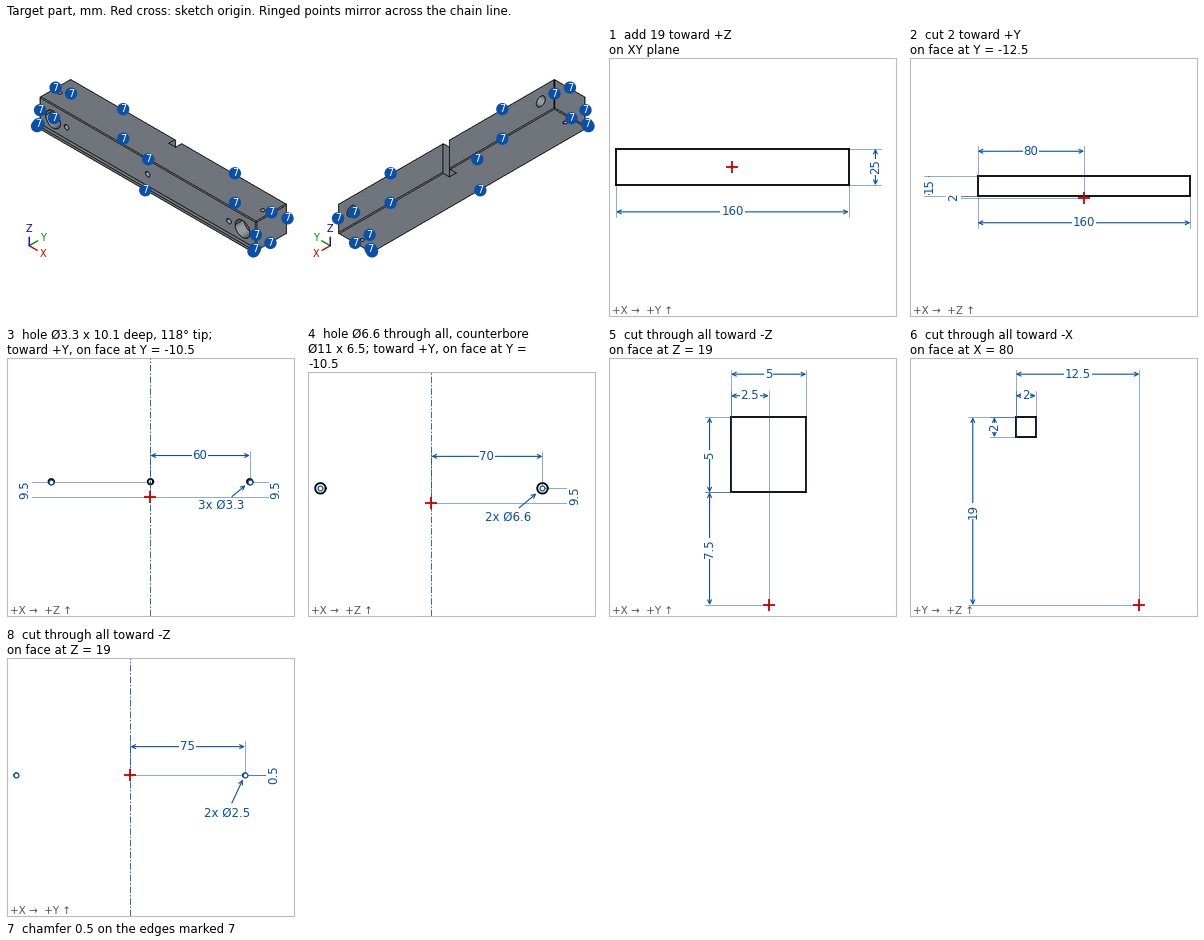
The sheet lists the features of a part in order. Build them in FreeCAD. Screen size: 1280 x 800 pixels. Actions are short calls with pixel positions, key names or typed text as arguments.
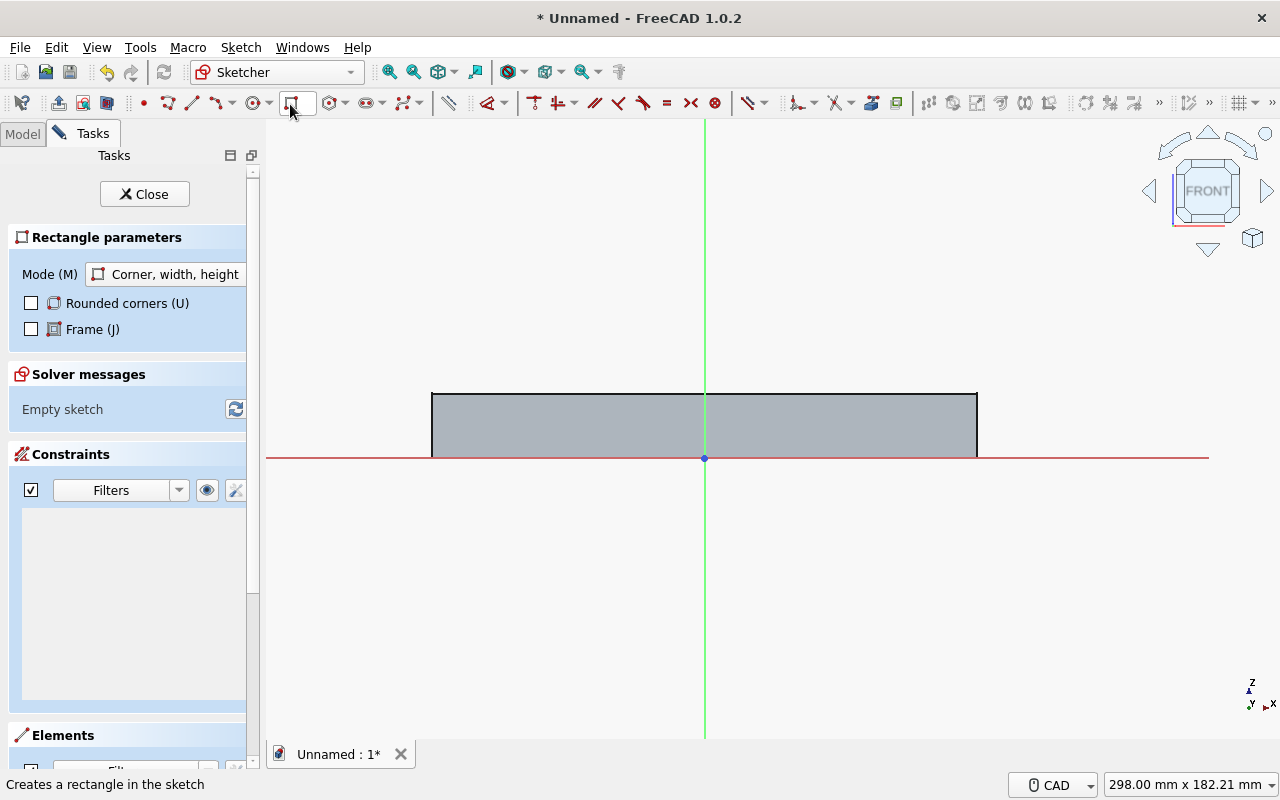
click(432, 400)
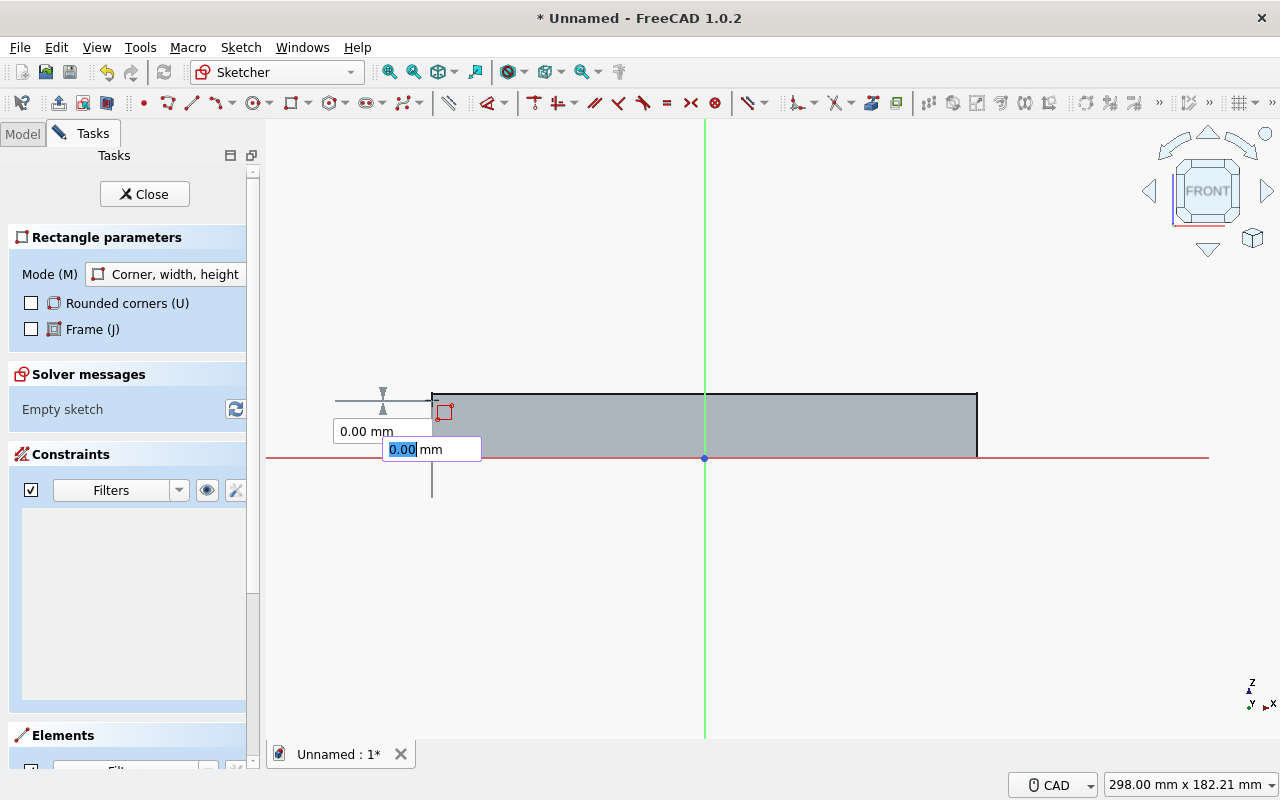
scroll(977, 451, up, 5)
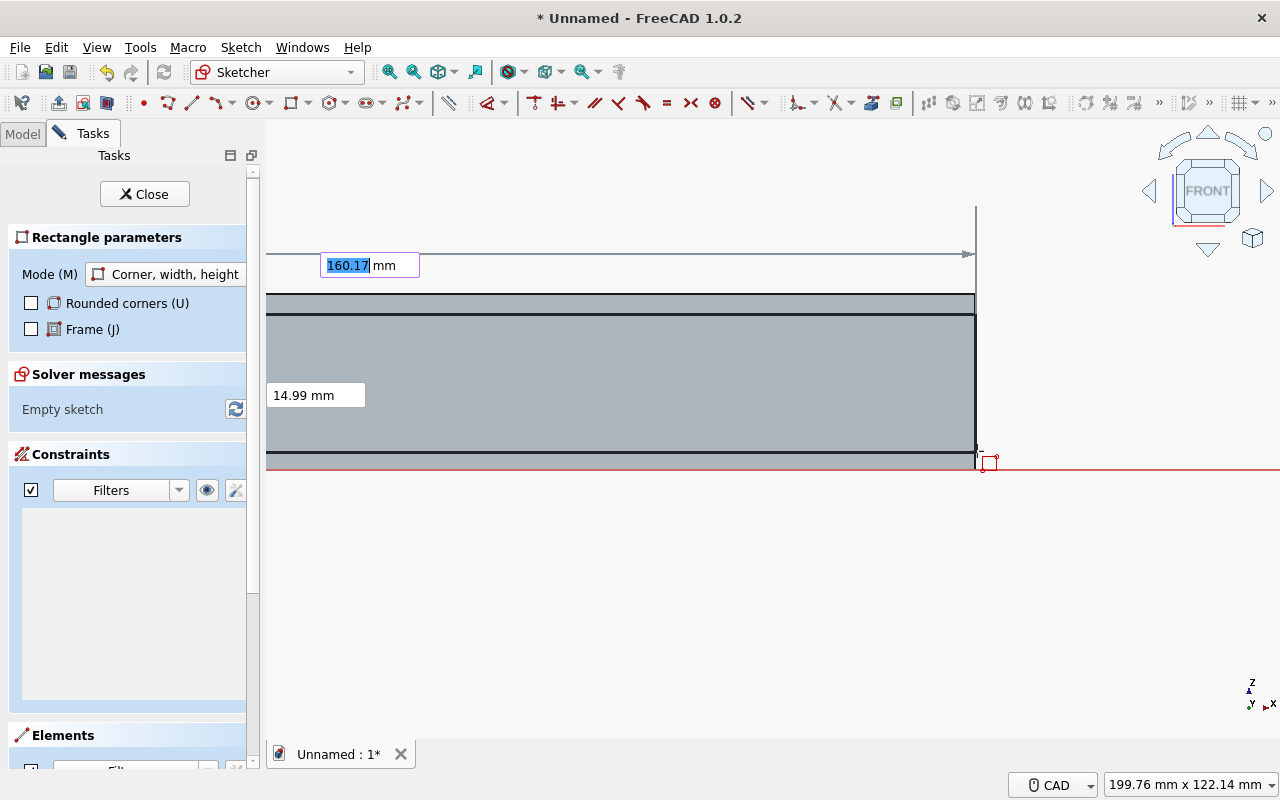
click(975, 451)
key(Escape)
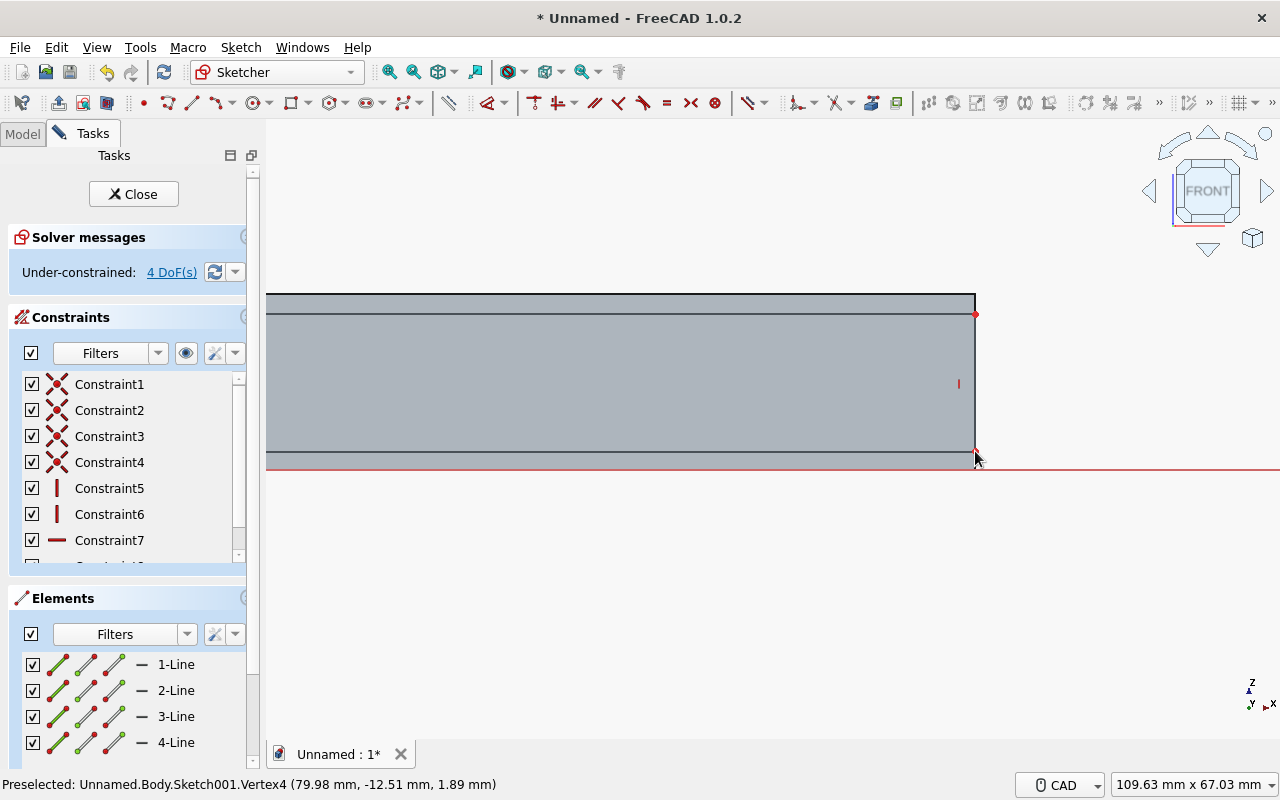
click(488, 104)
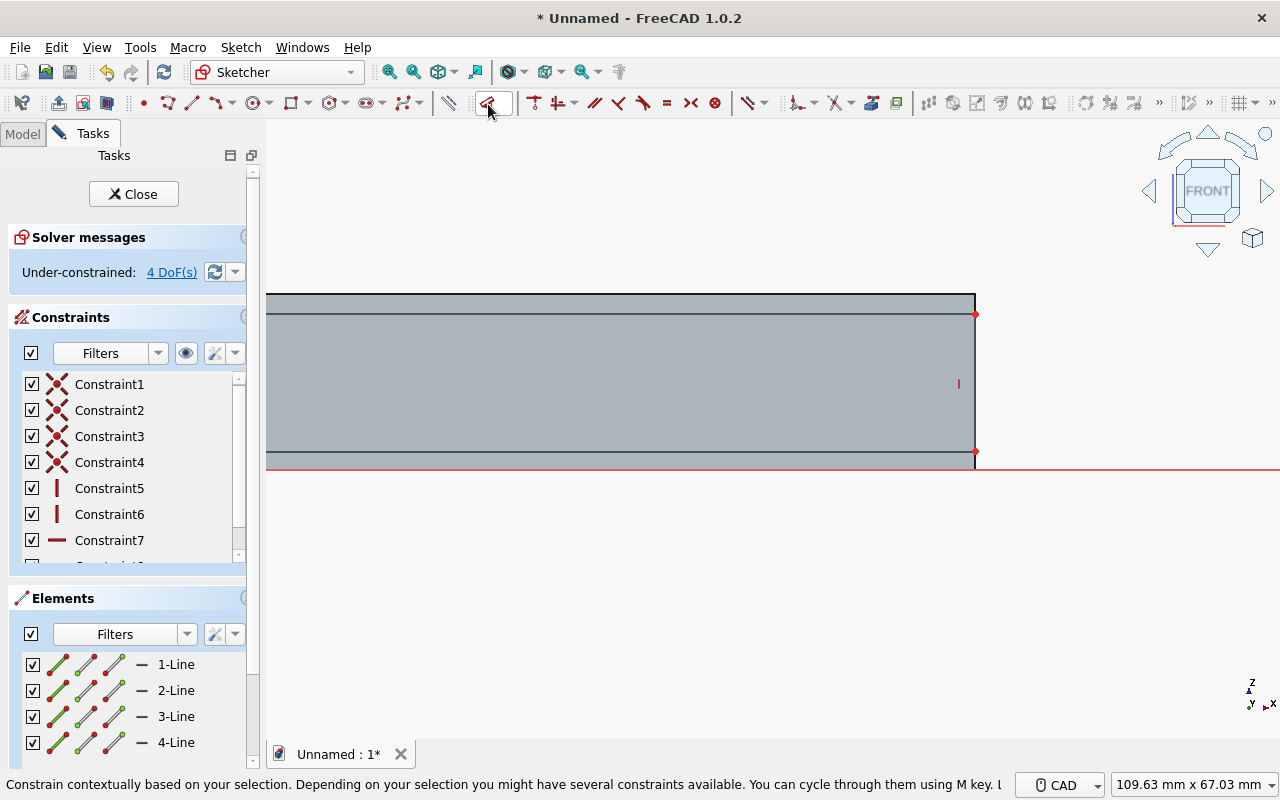
scroll(978, 451, down, 5)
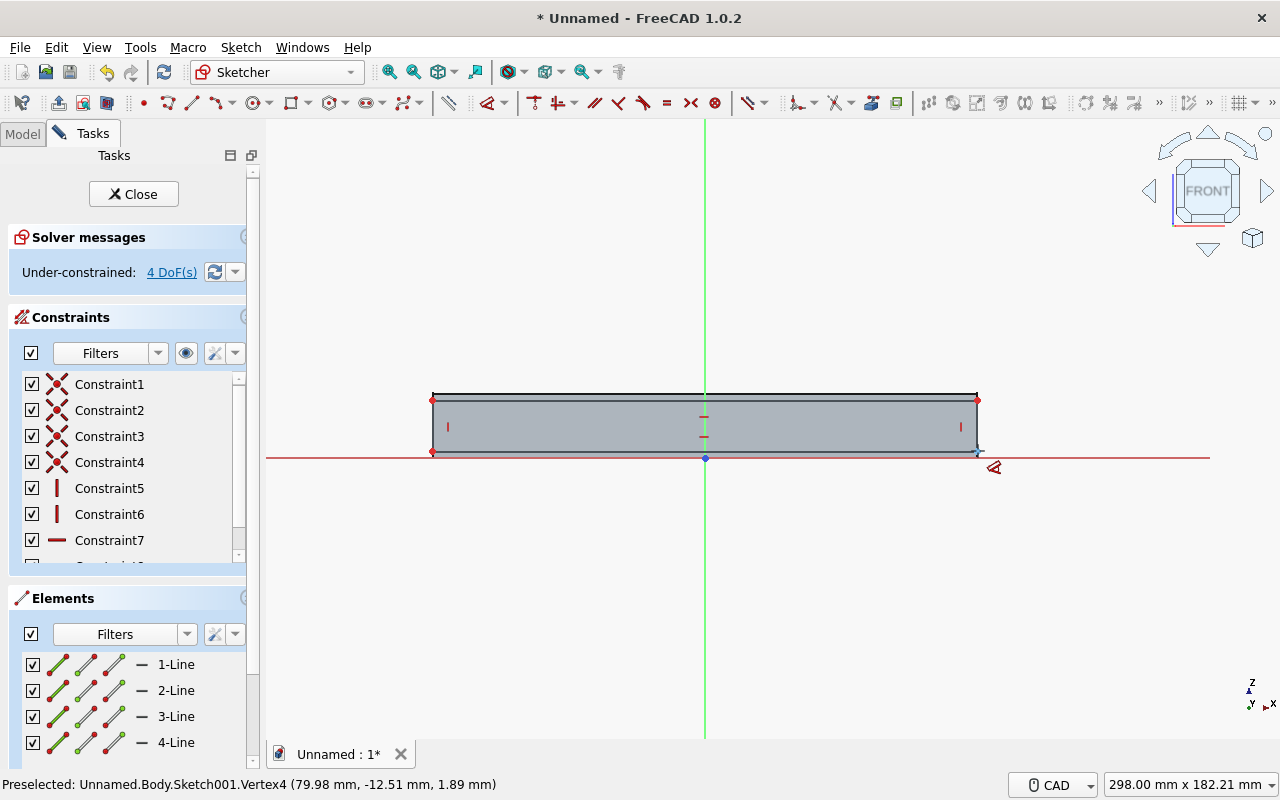
click(433, 416)
click(399, 426)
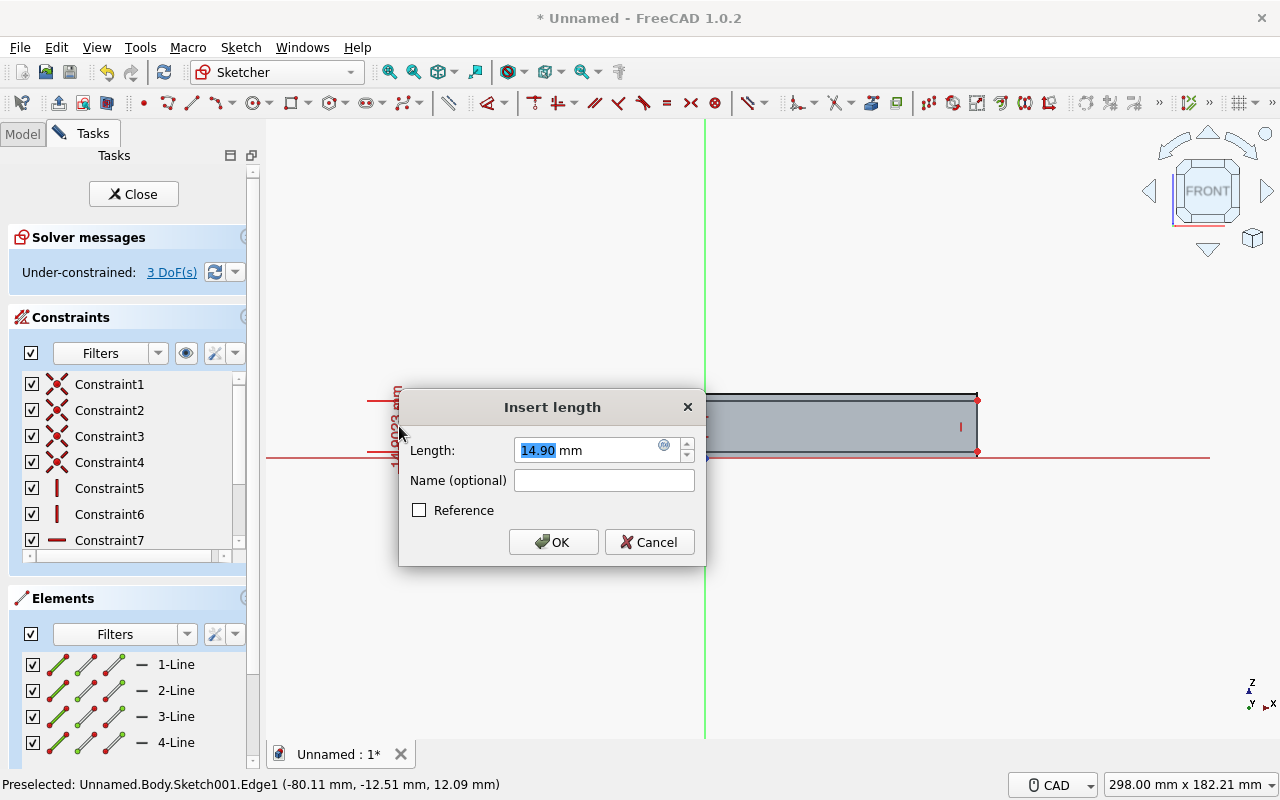
text(15)
key(Return)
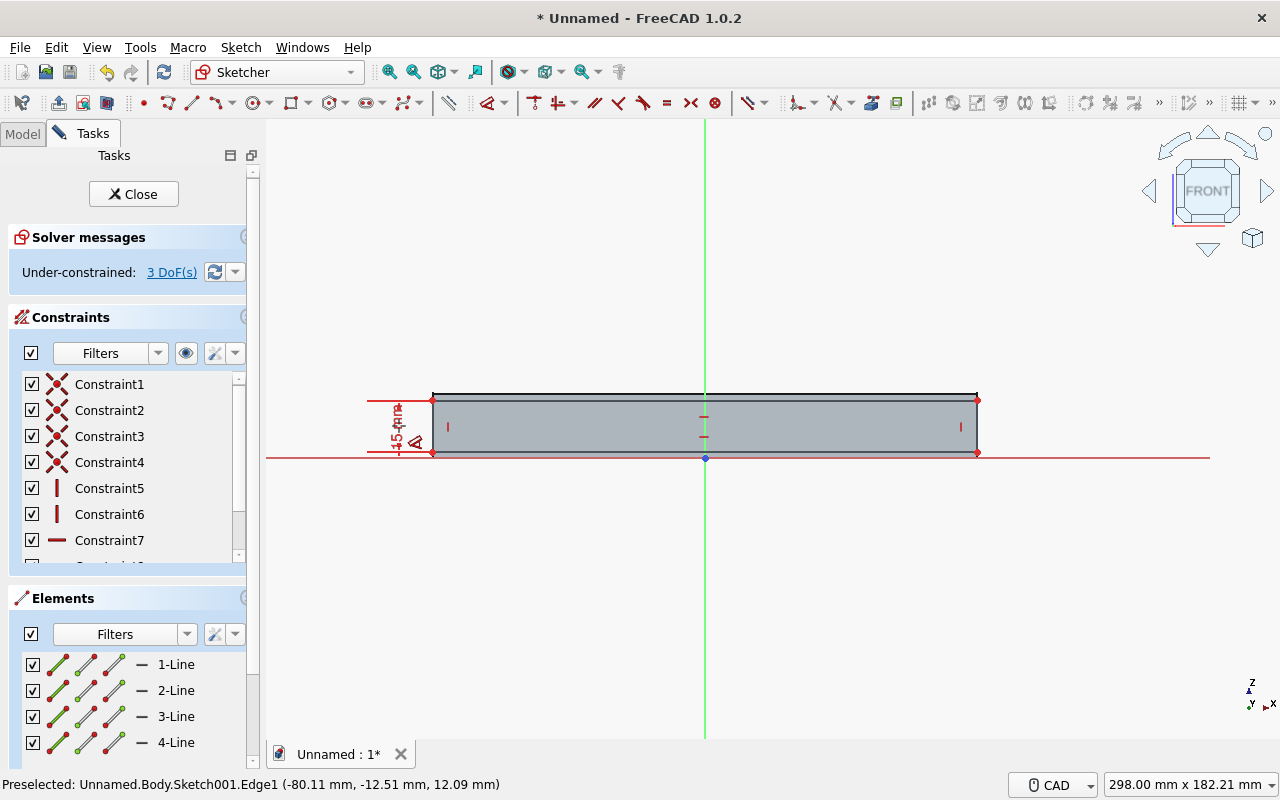
scroll(433, 452, up, 9)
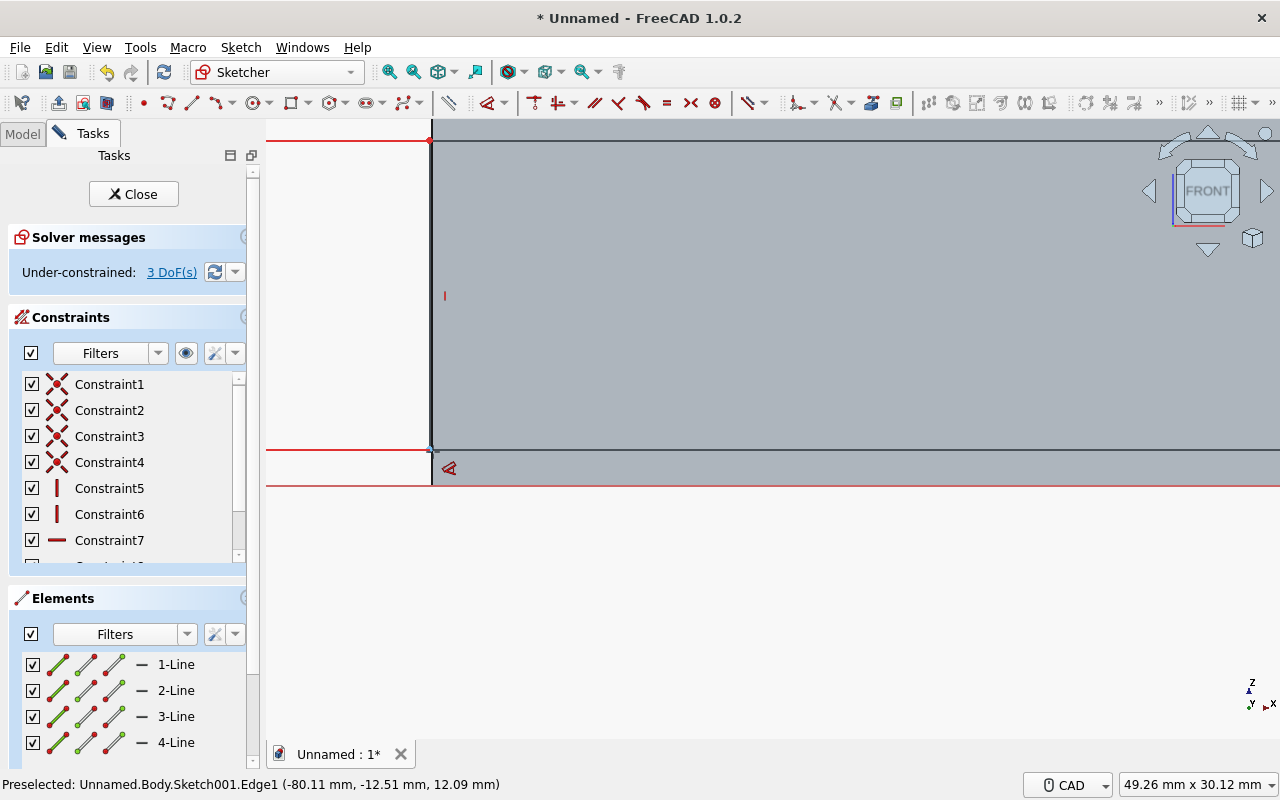
click(430, 450)
click(396, 468)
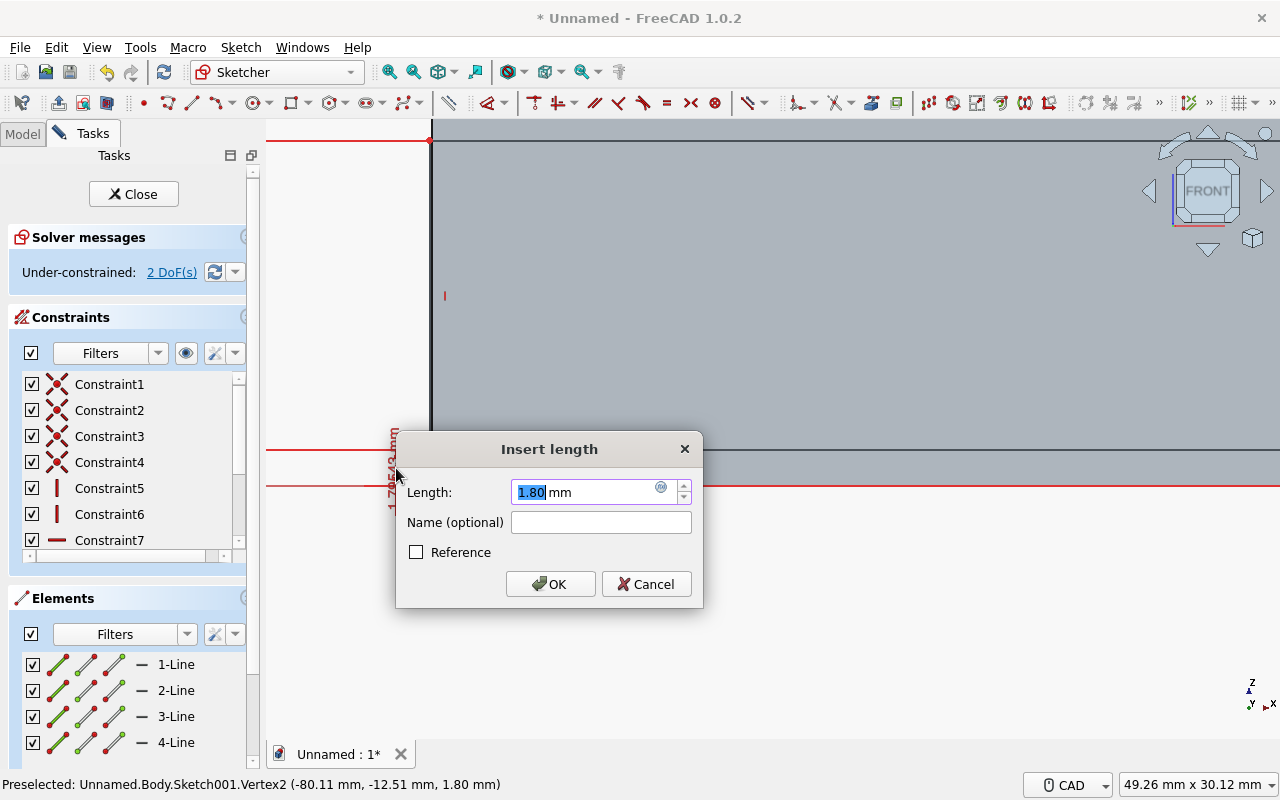
text(2)
key(Return)